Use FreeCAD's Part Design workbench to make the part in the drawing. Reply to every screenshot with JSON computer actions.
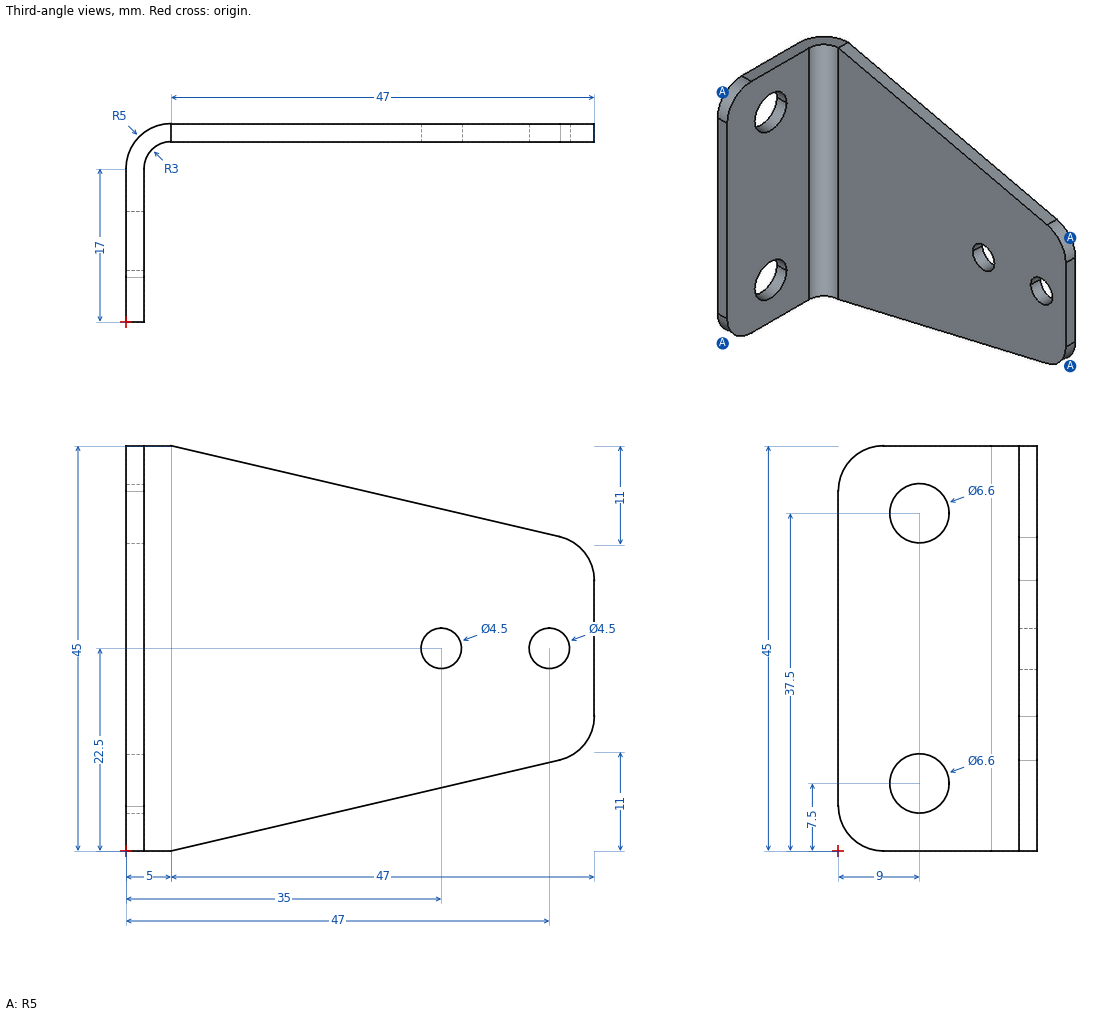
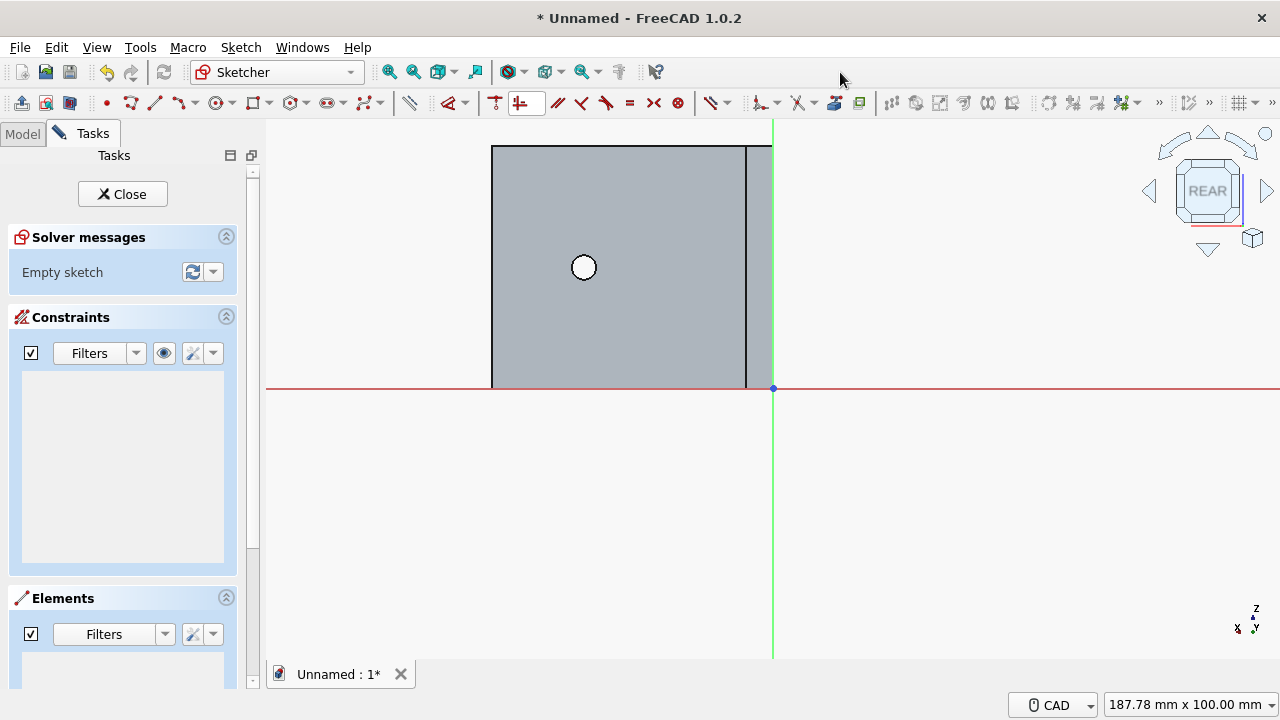
{"action": "scroll", "coordinate": [504, 258], "scroll_direction": "up", "scroll_amount": 13}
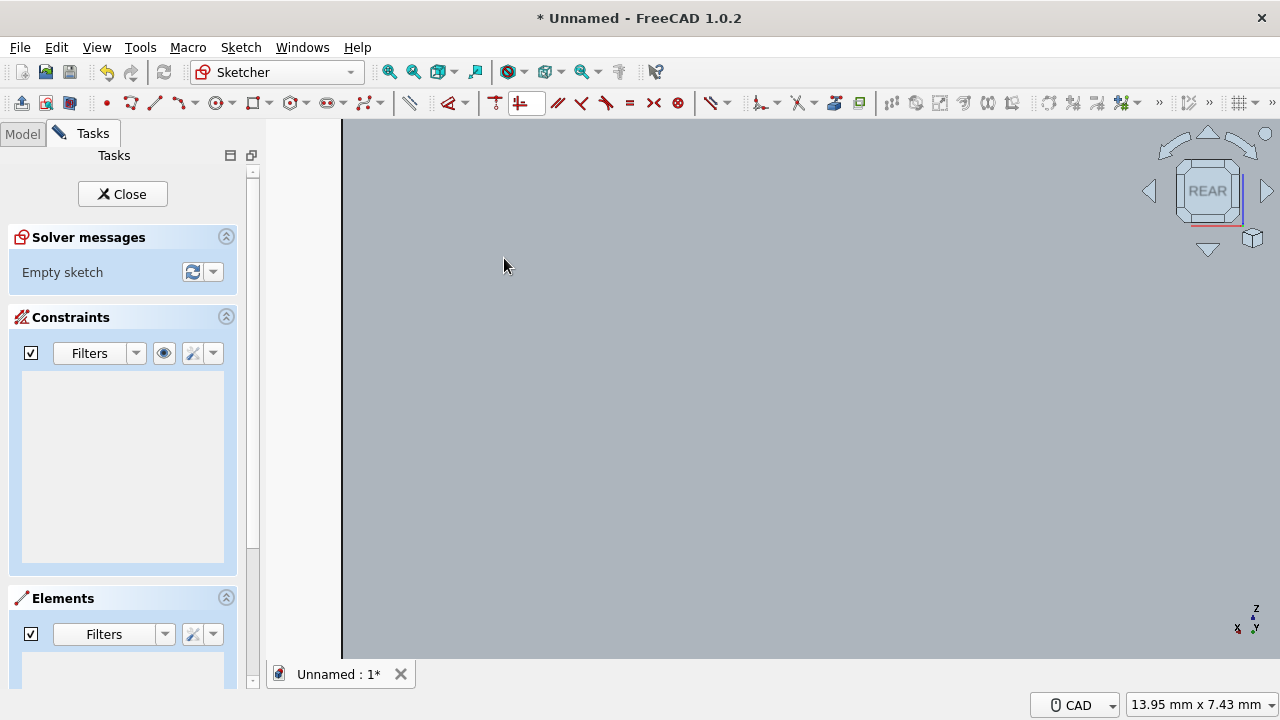
{"action": "key", "text": "g c"}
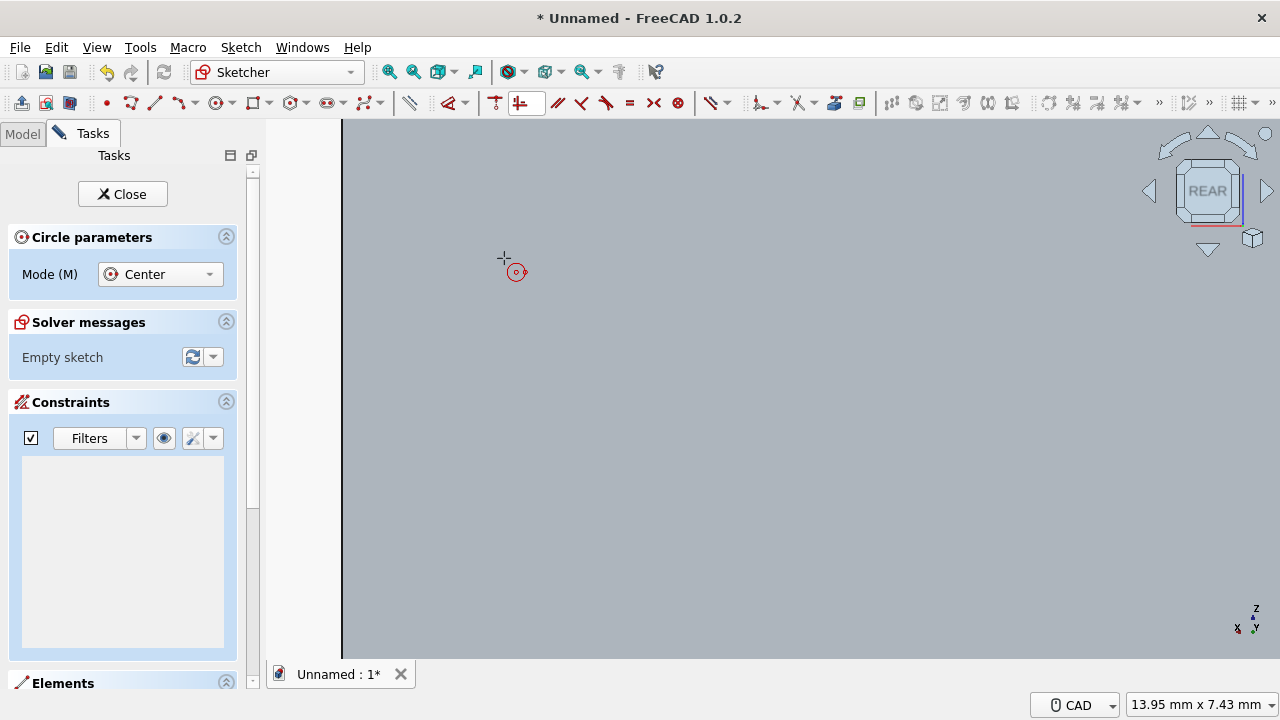
{"action": "left_click", "coordinate": [706, 383]}
{"action": "mouse_move", "coordinate": [821, 267]}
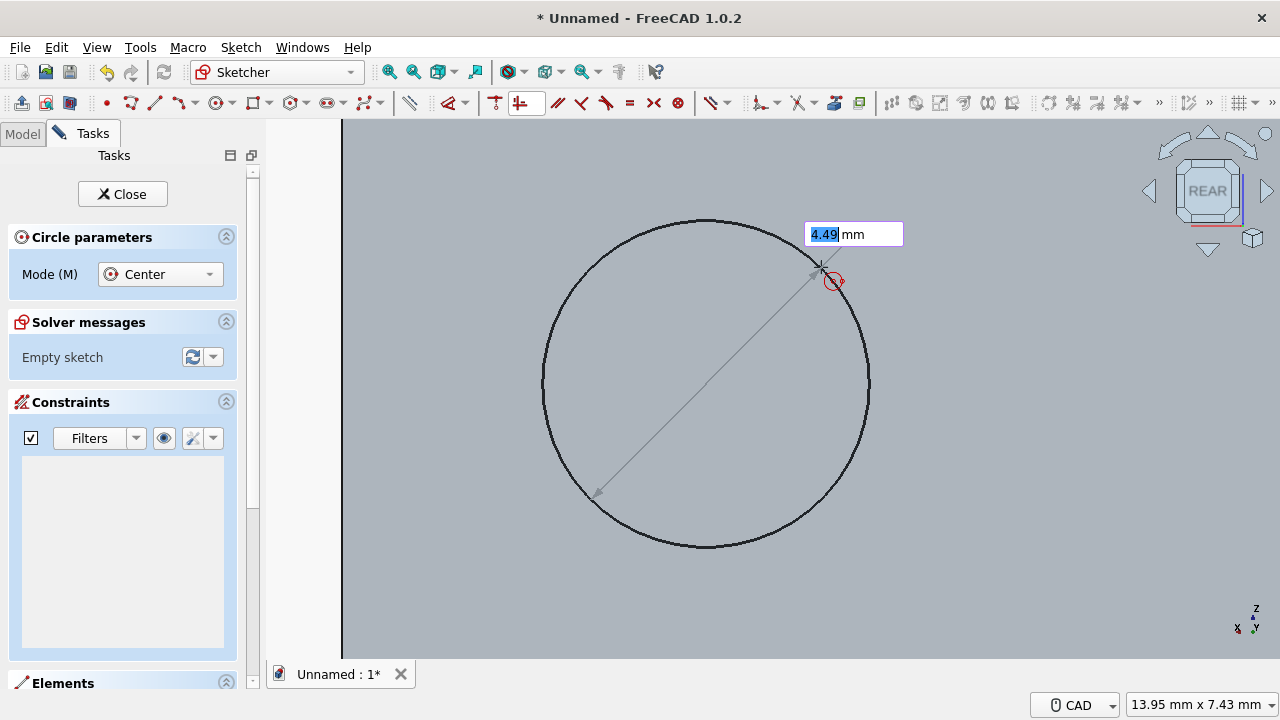
{"action": "type", "text": "4.5"}
{"action": "key", "text": "Return"}
{"action": "key", "text": "Escape"}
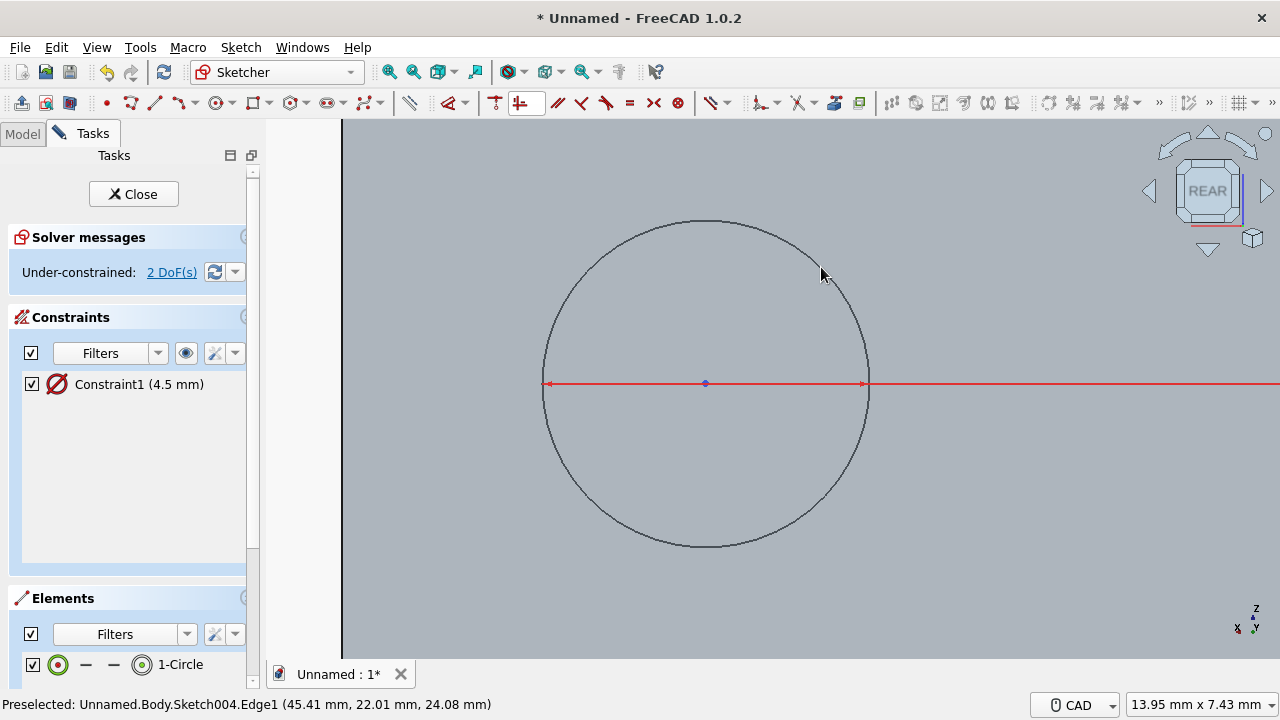
{"action": "key", "text": "d"}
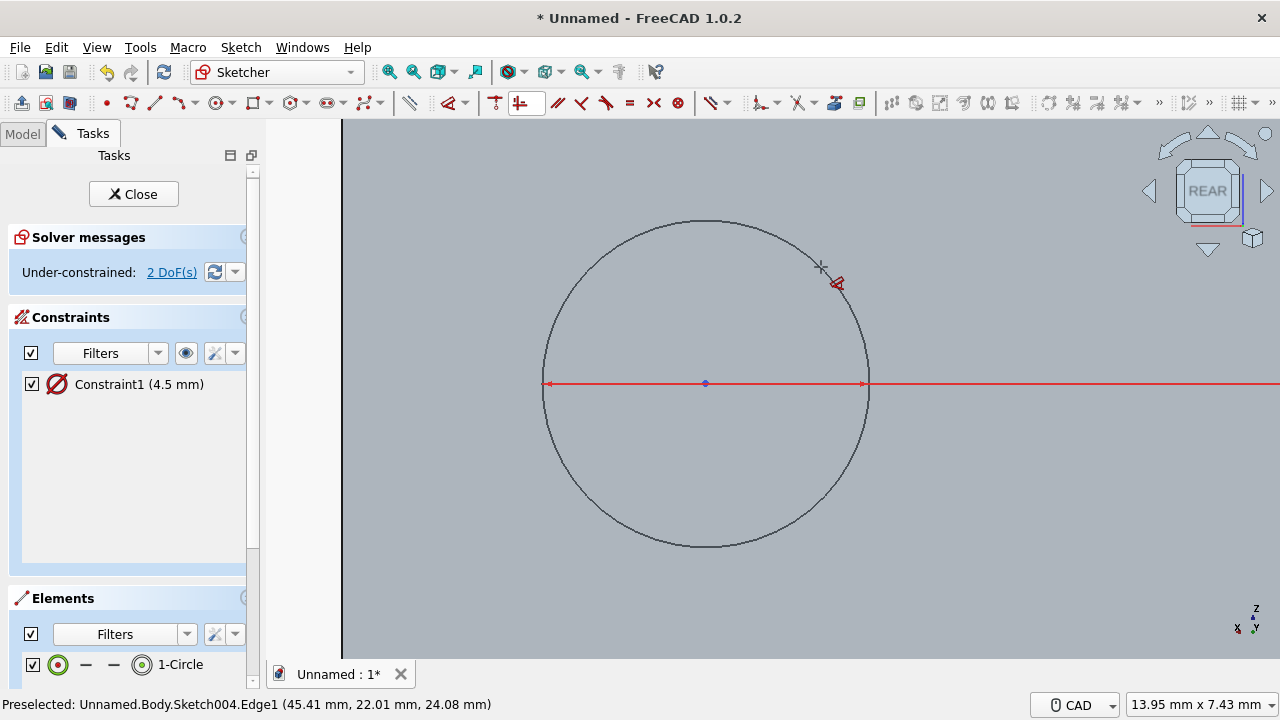
{"action": "left_click", "coordinate": [706, 384]}
{"action": "left_click", "coordinate": [910, 350]}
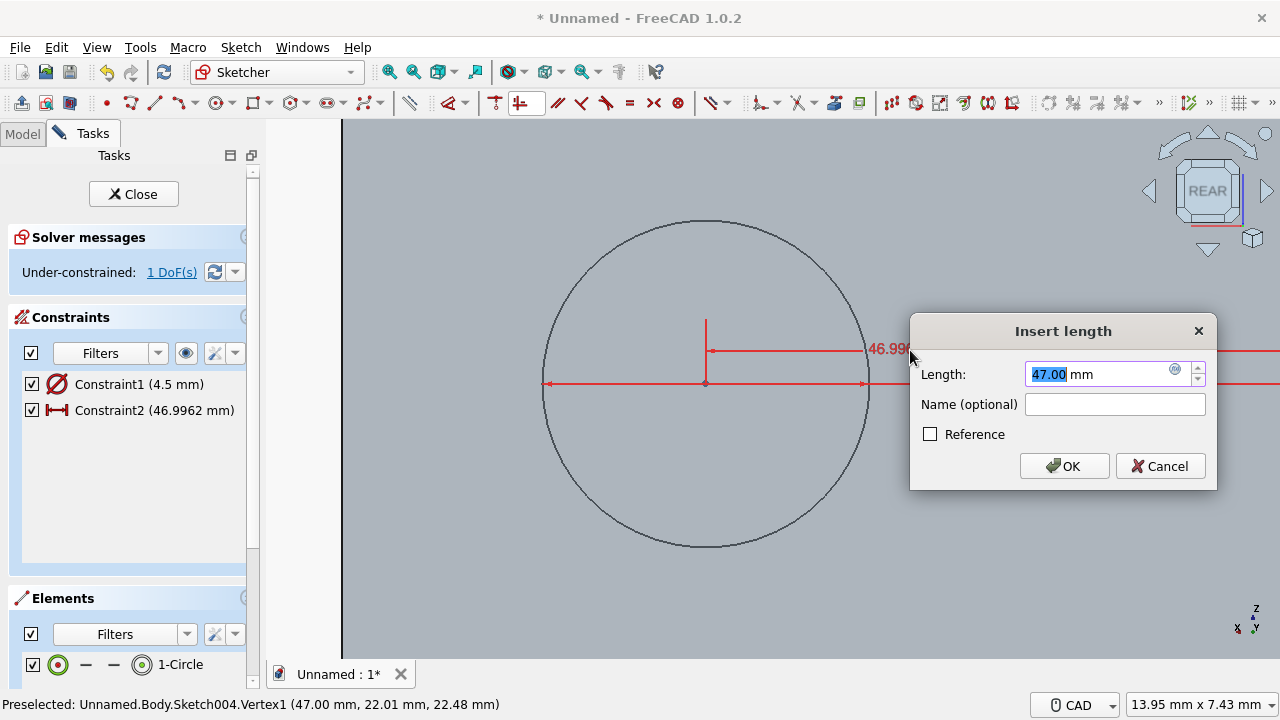
{"action": "type", "text": "47"}
{"action": "key", "text": "Return"}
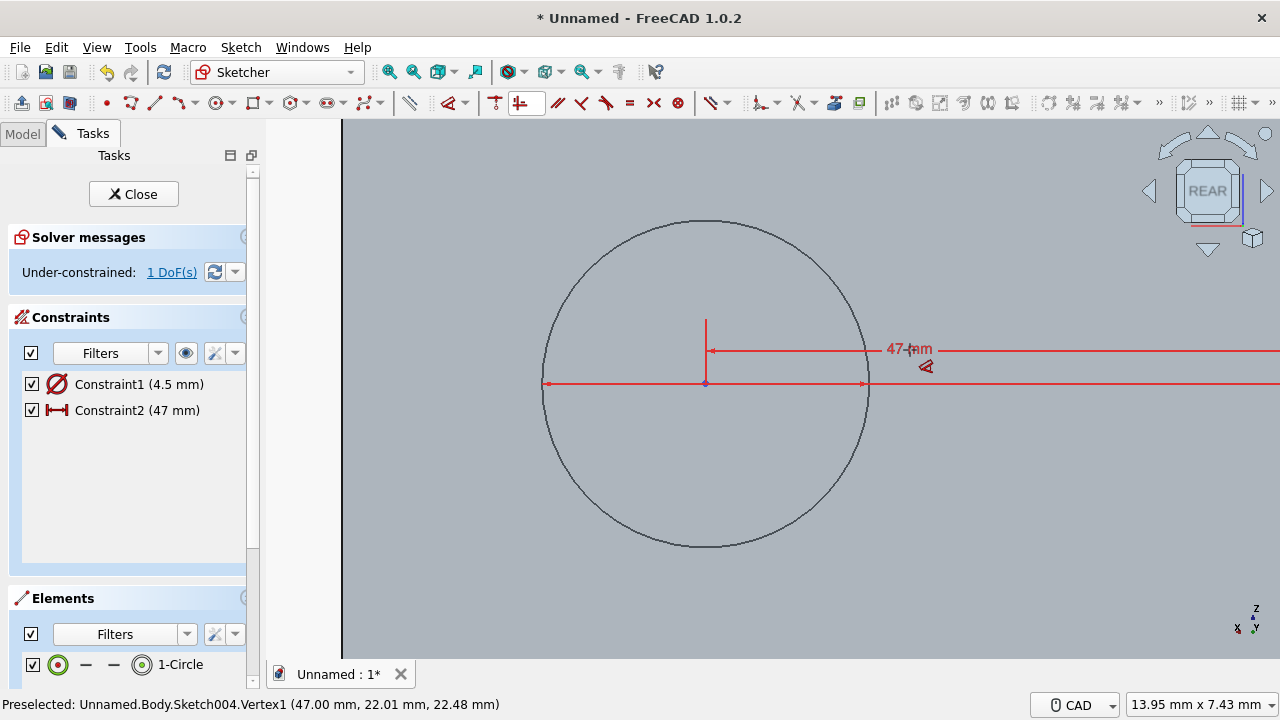
{"action": "left_click", "coordinate": [706, 384]}
{"action": "left_click", "coordinate": [672, 508]}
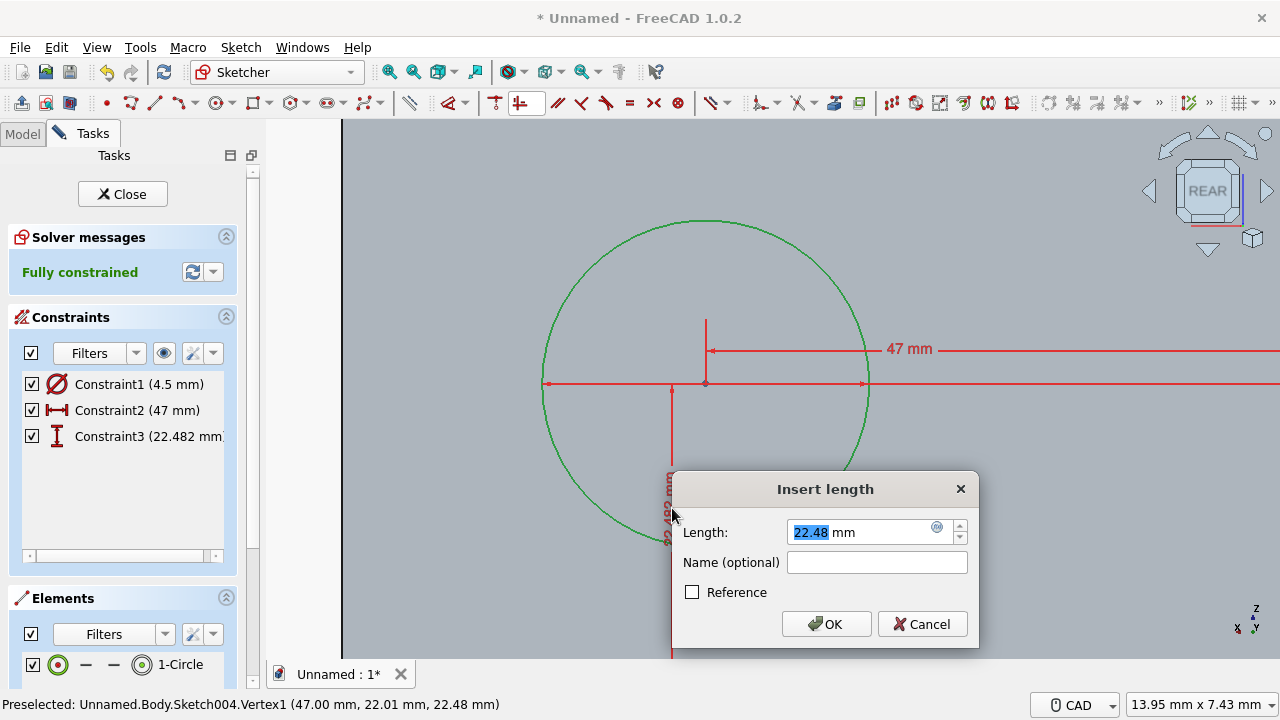
{"action": "type", "text": "22.5"}
{"action": "key", "text": "Return"}
{"action": "key", "text": "Escape"}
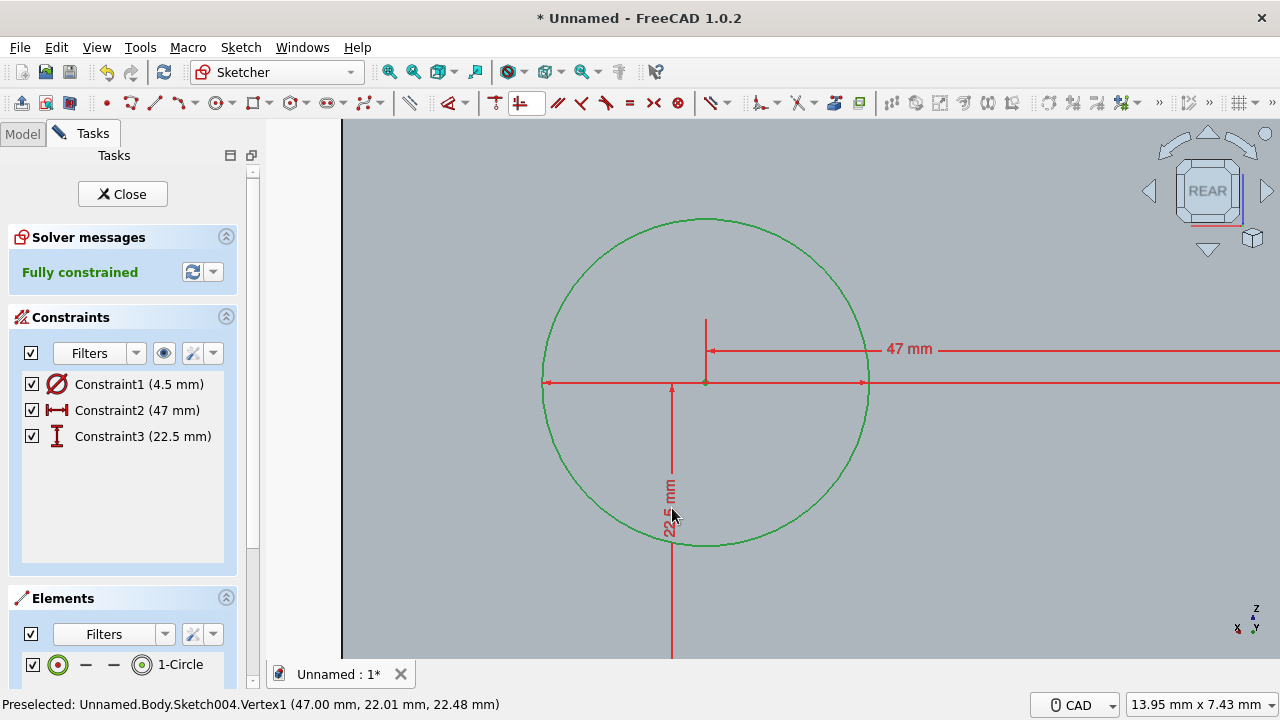
{"action": "left_click", "coordinate": [123, 194]}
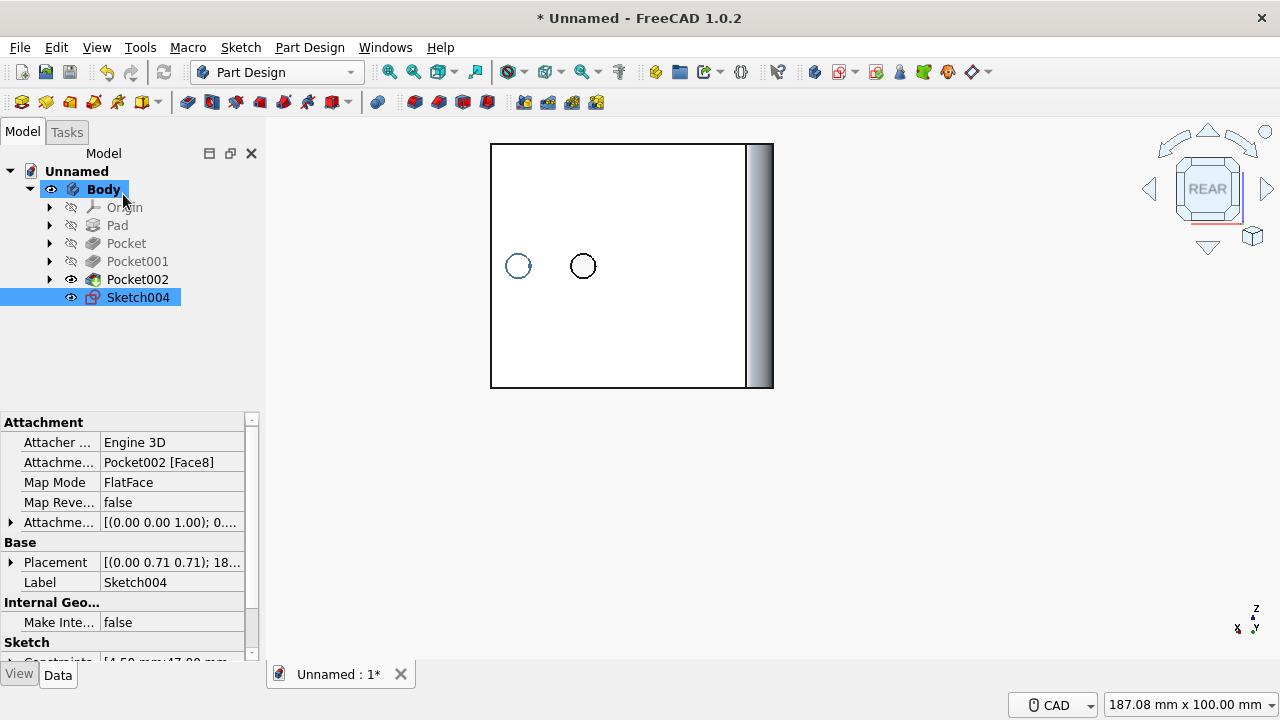
{"action": "left_click", "coordinate": [188, 102]}